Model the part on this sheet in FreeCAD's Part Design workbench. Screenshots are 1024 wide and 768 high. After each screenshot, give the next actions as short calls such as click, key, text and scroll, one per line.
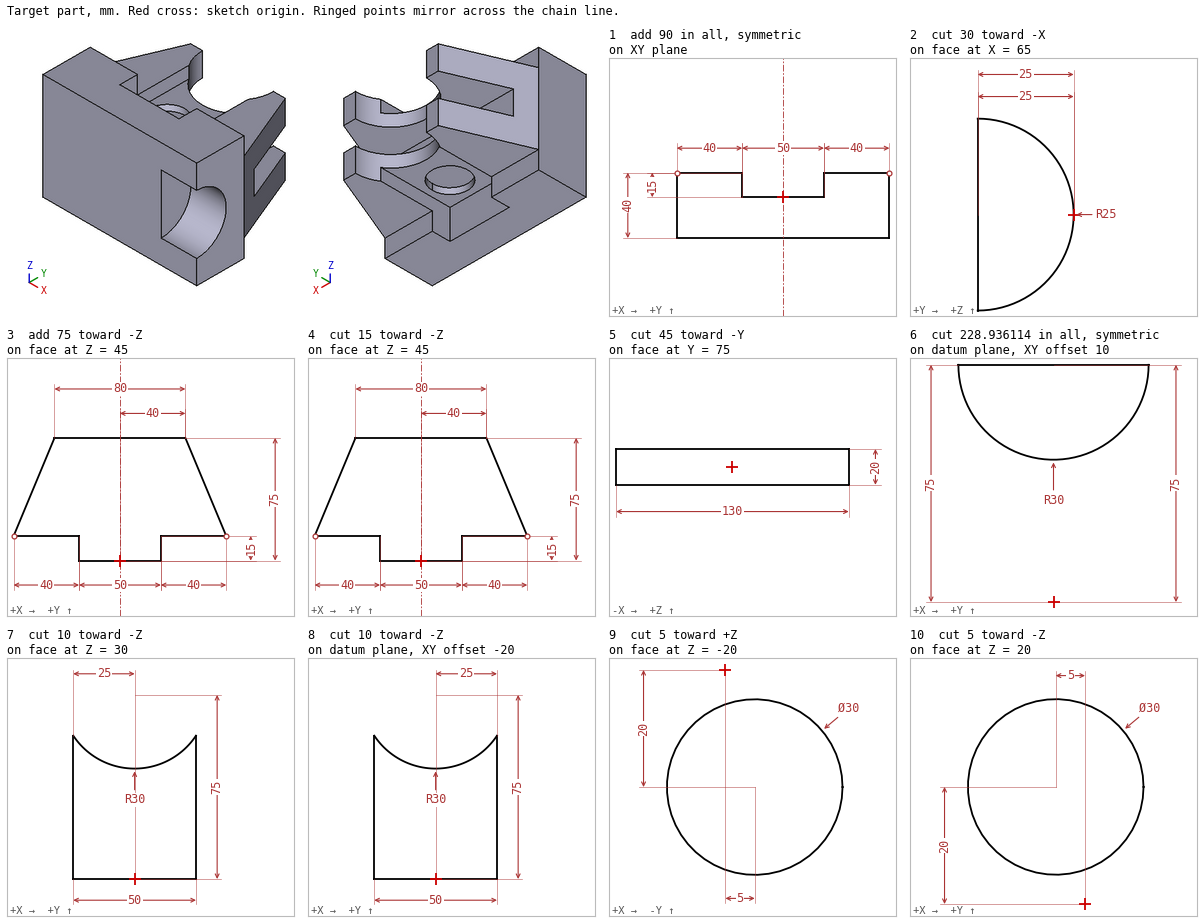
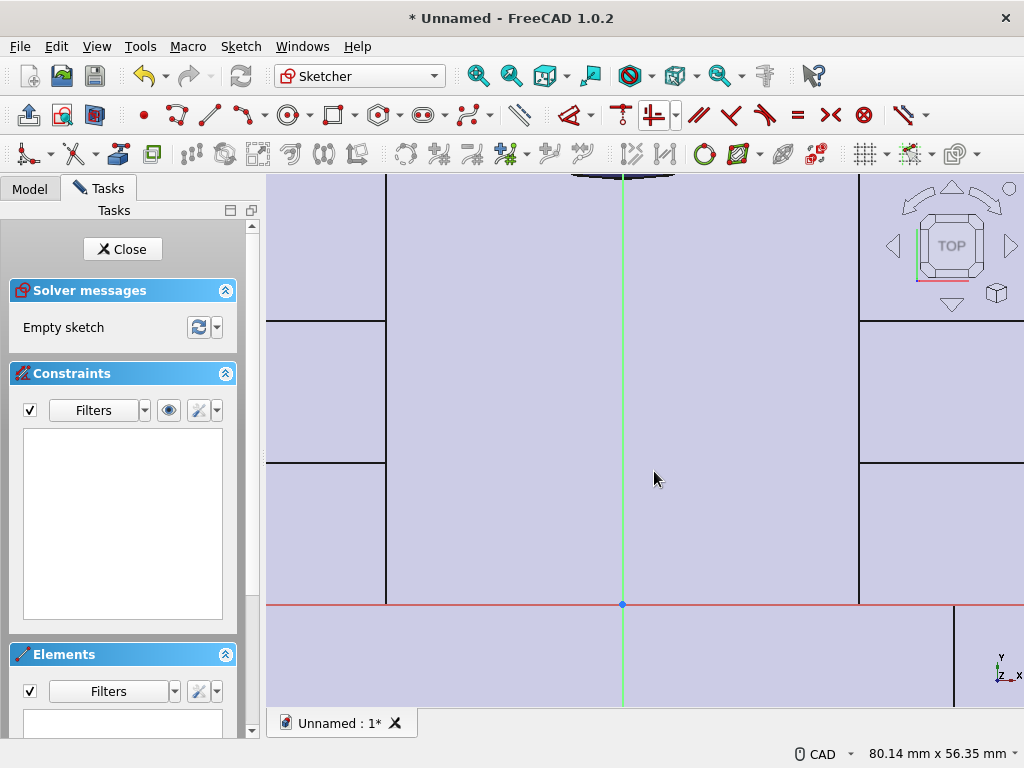
click(288, 116)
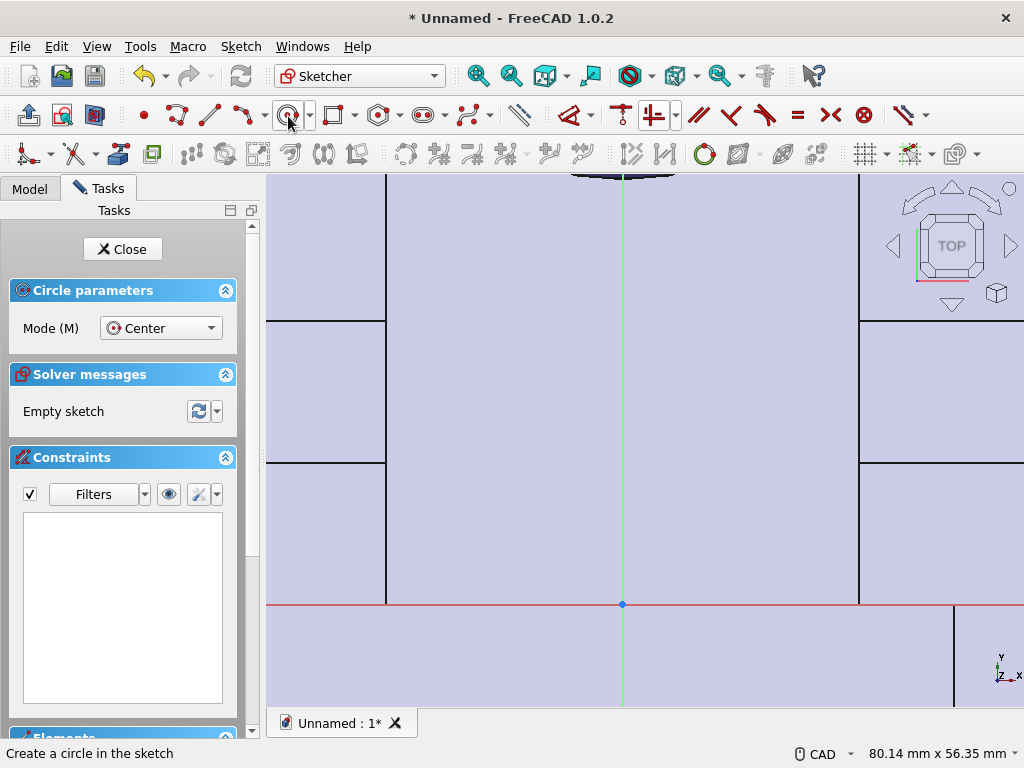
click(576, 416)
click(676, 315)
key(Escape)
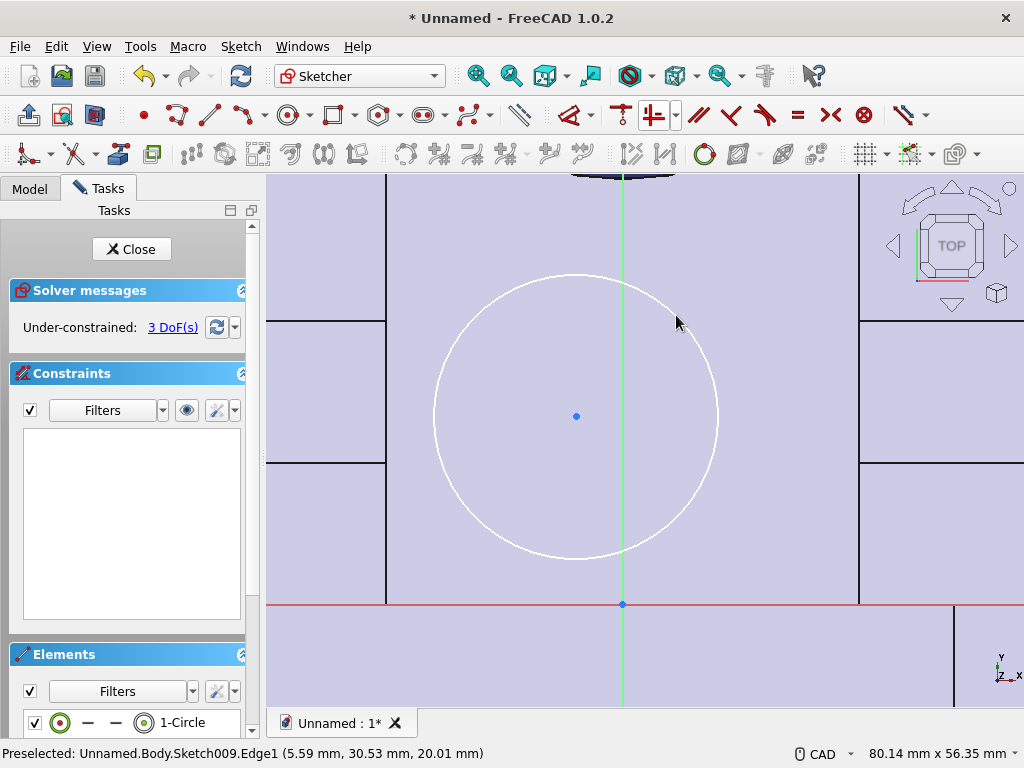
click(568, 116)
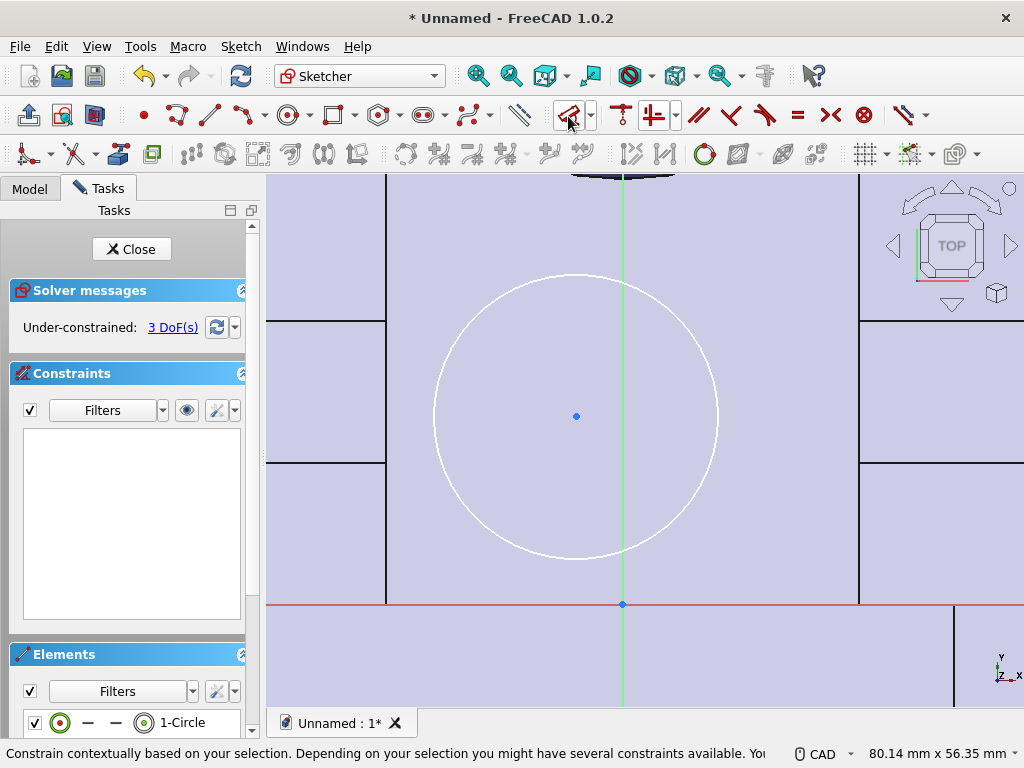
click(676, 316)
click(699, 293)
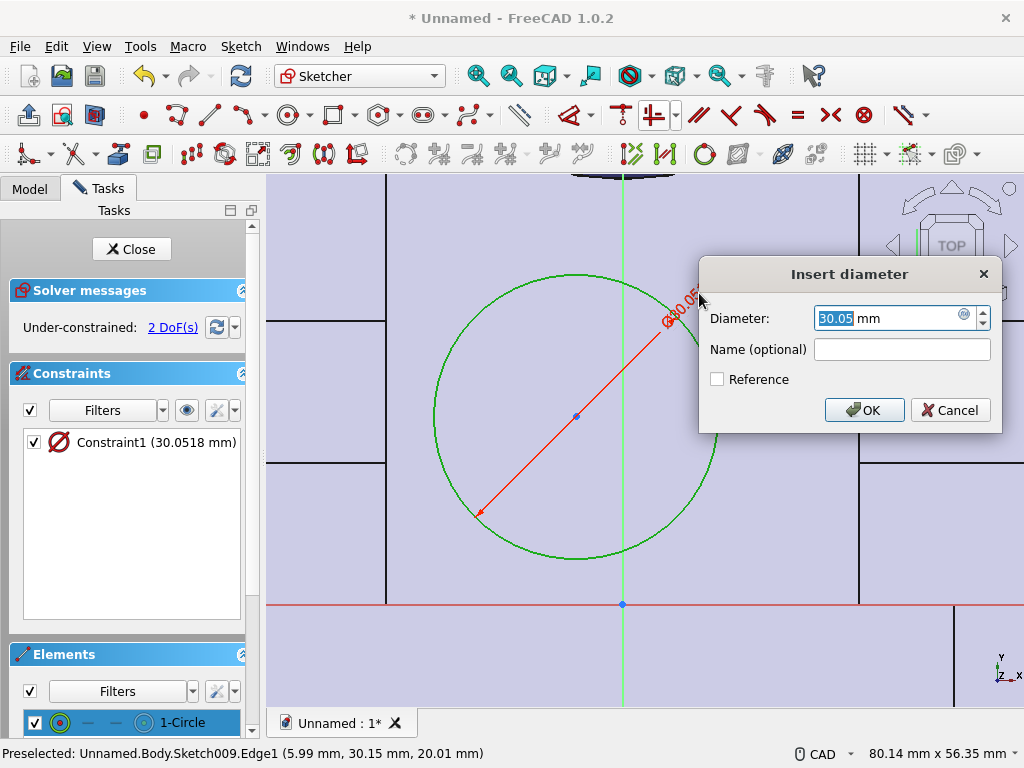
text(30)
key(Return)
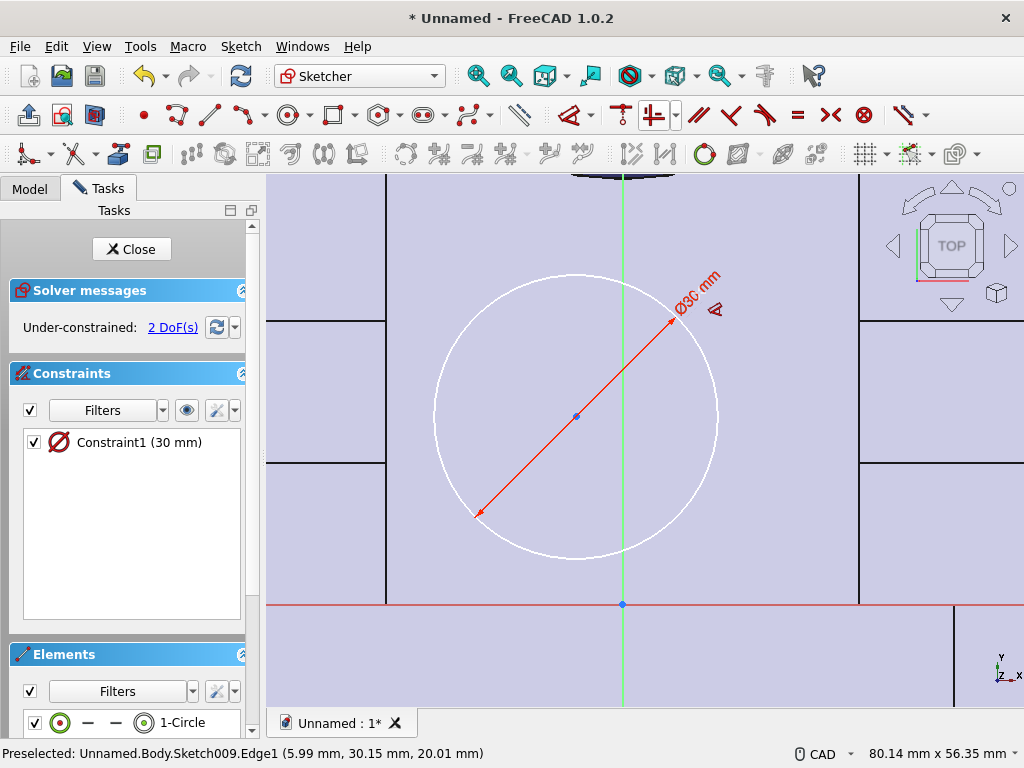
click(576, 417)
click(599, 639)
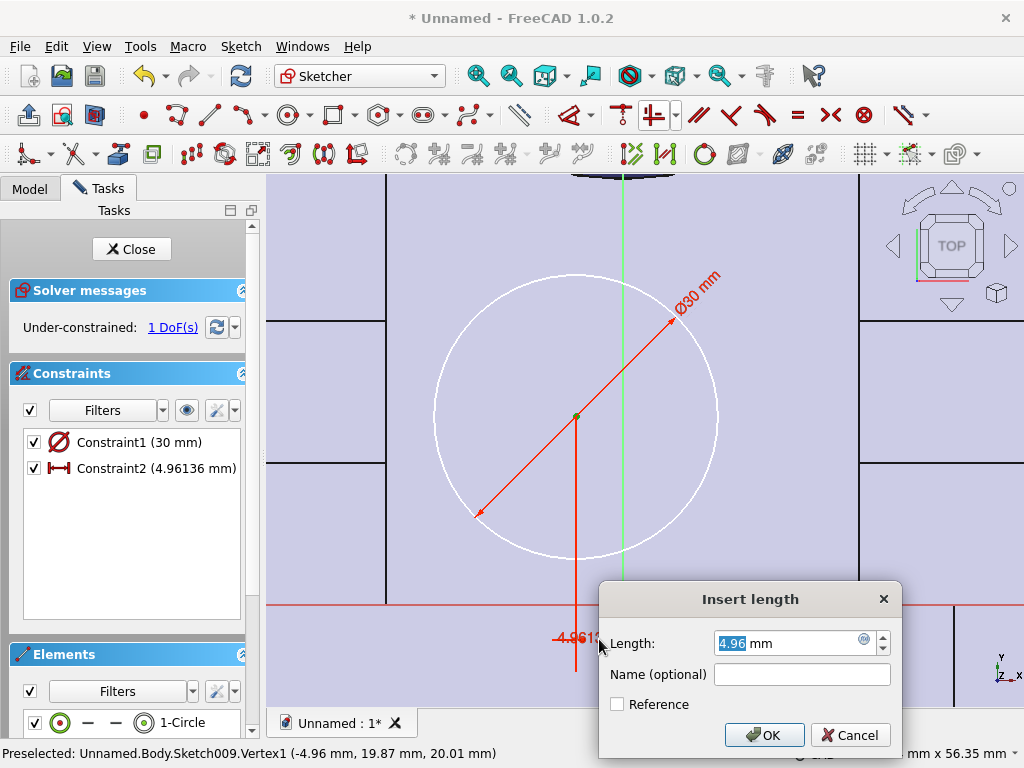
text(5)
key(Return)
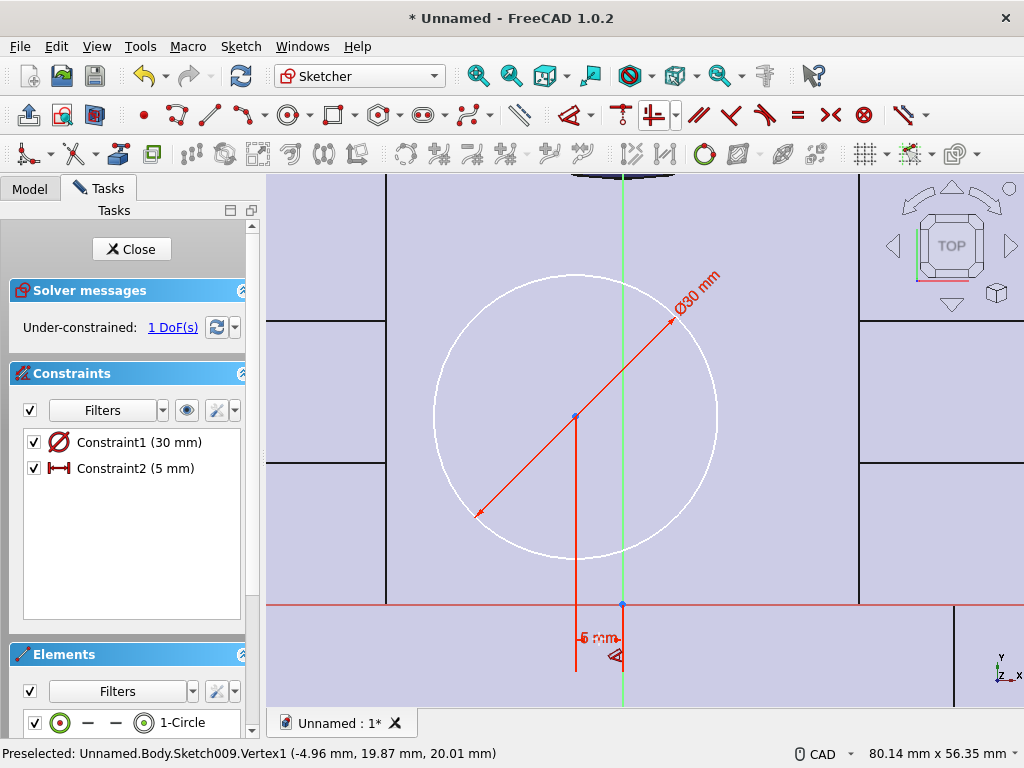
click(576, 417)
click(657, 511)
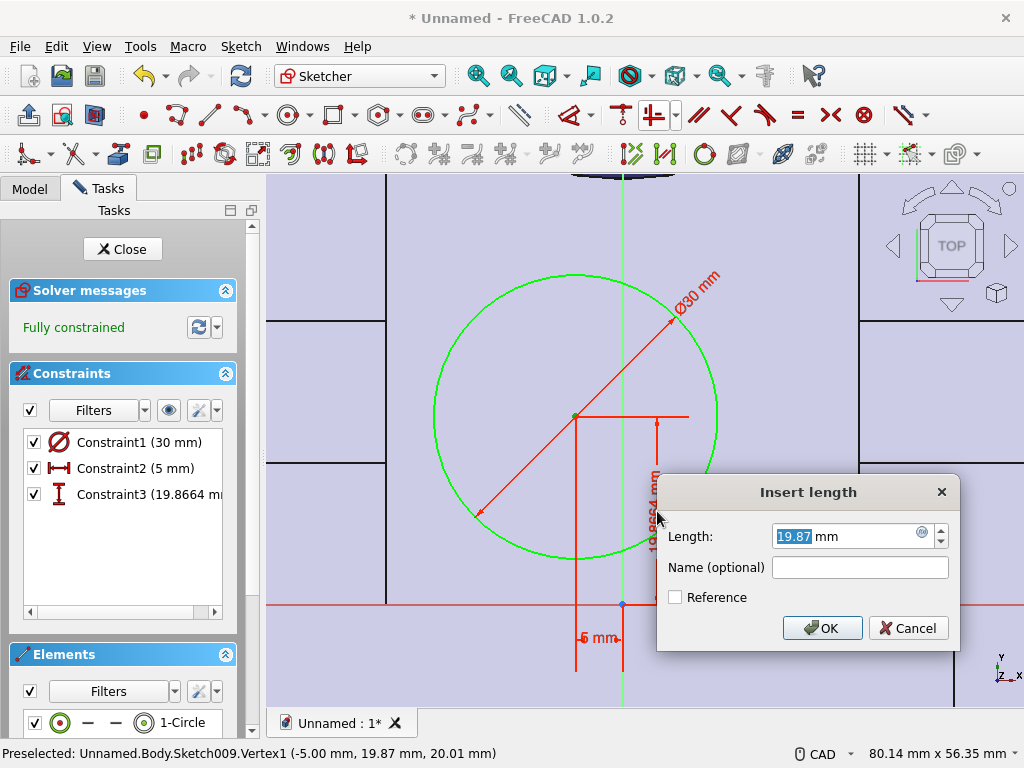
text(20)
key(Return)
key(Escape)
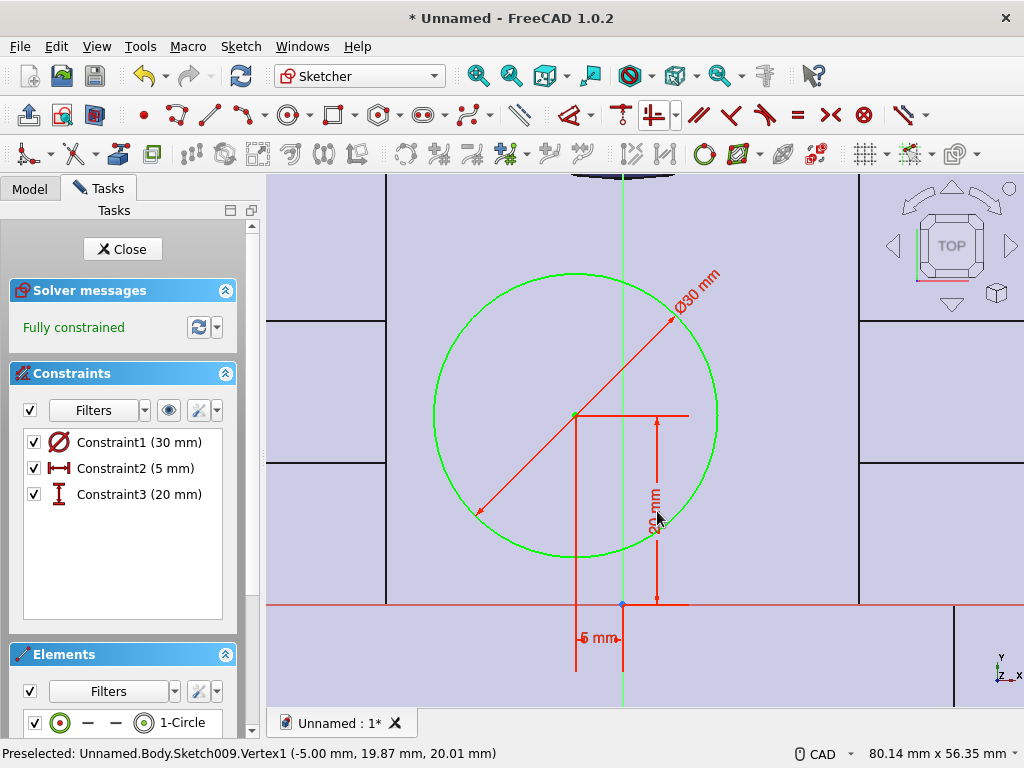
click(123, 249)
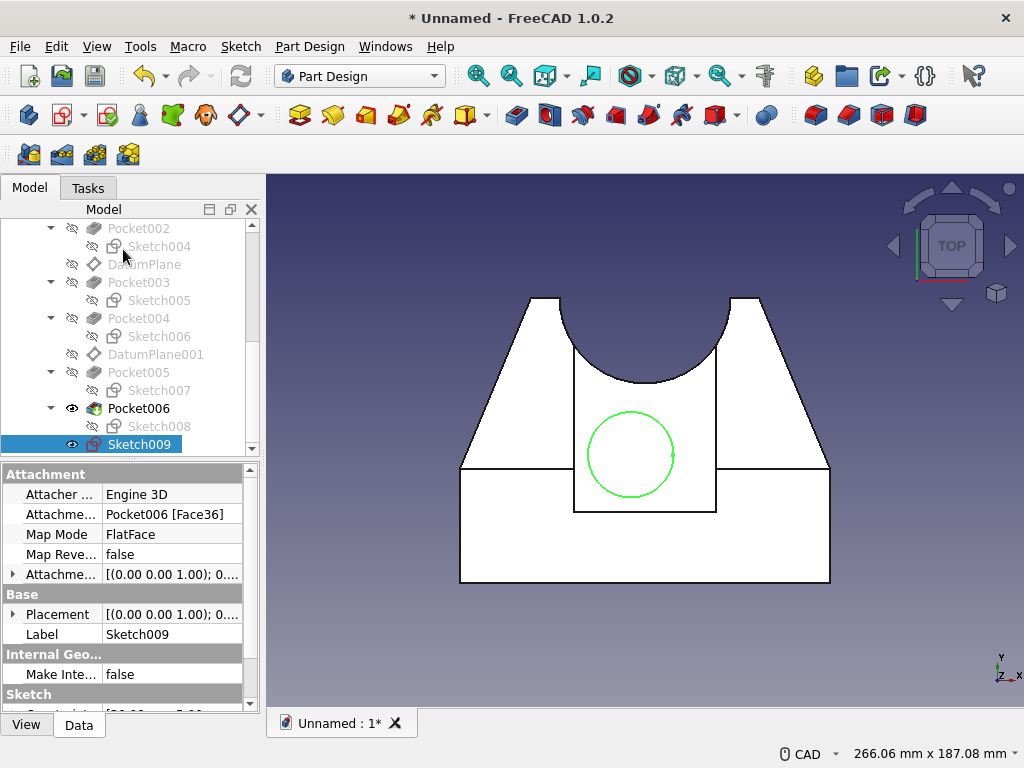
click(517, 116)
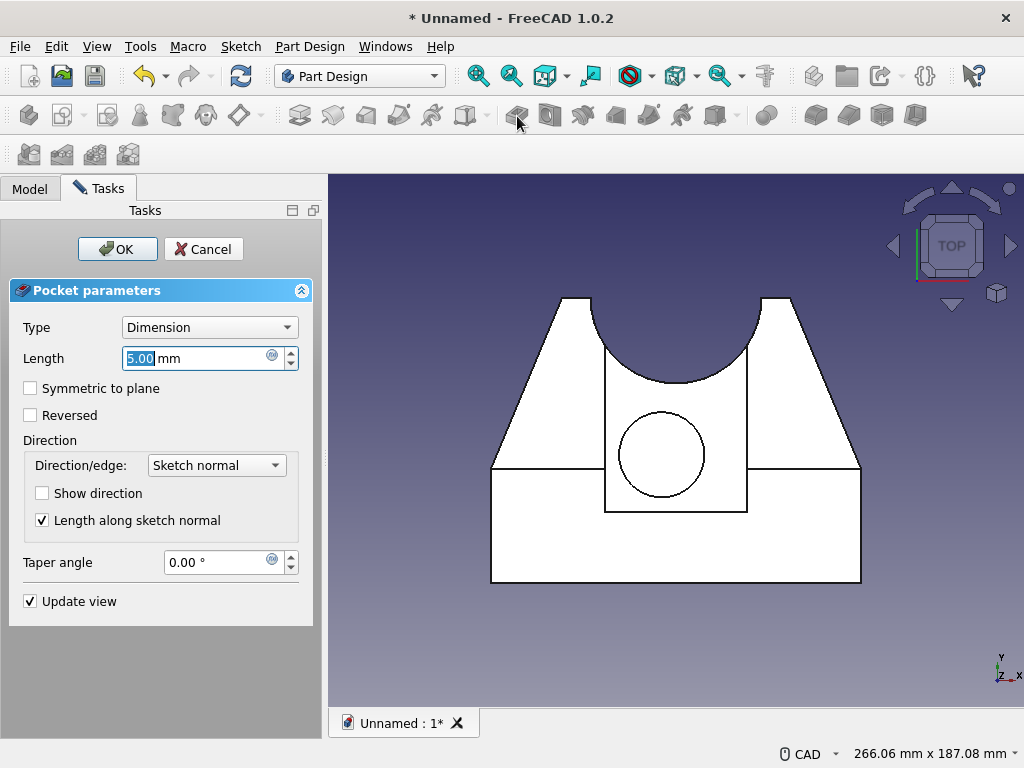
text(5)
key(Tab)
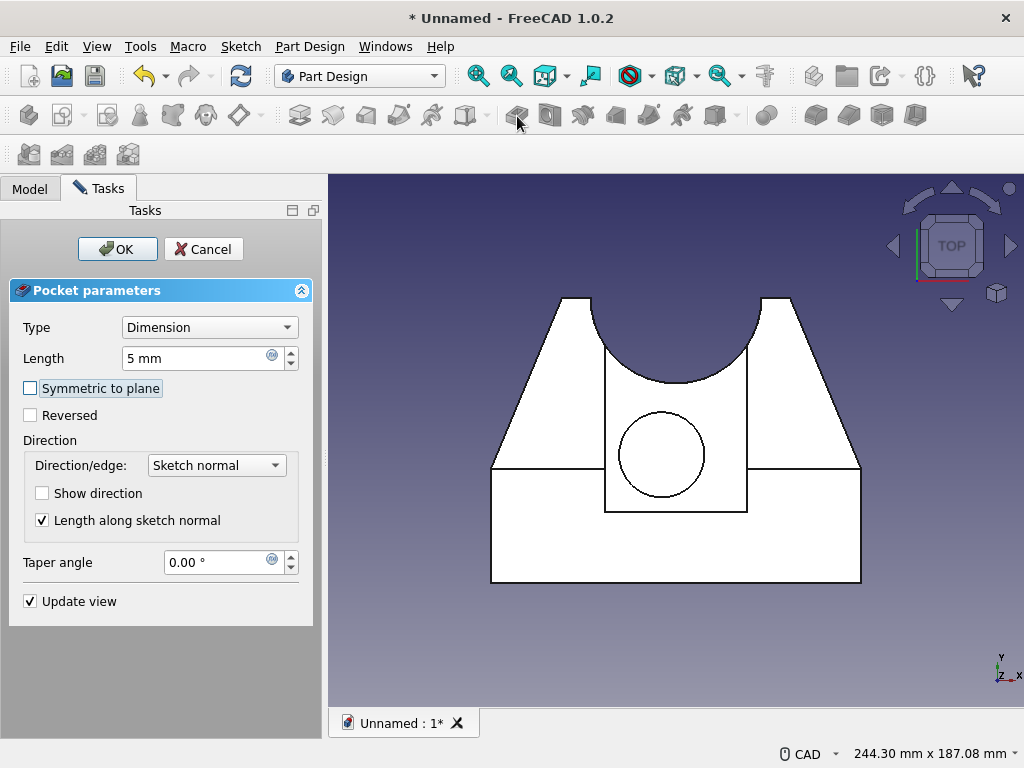
click(118, 249)